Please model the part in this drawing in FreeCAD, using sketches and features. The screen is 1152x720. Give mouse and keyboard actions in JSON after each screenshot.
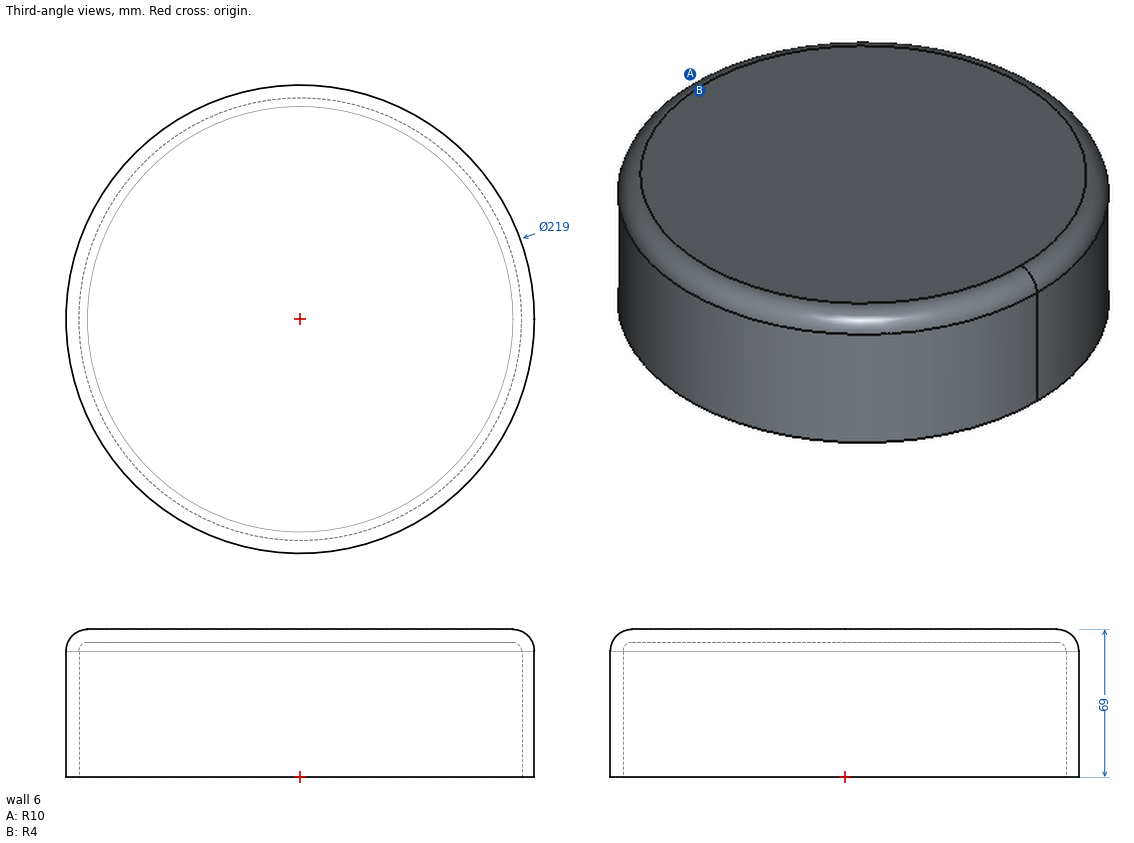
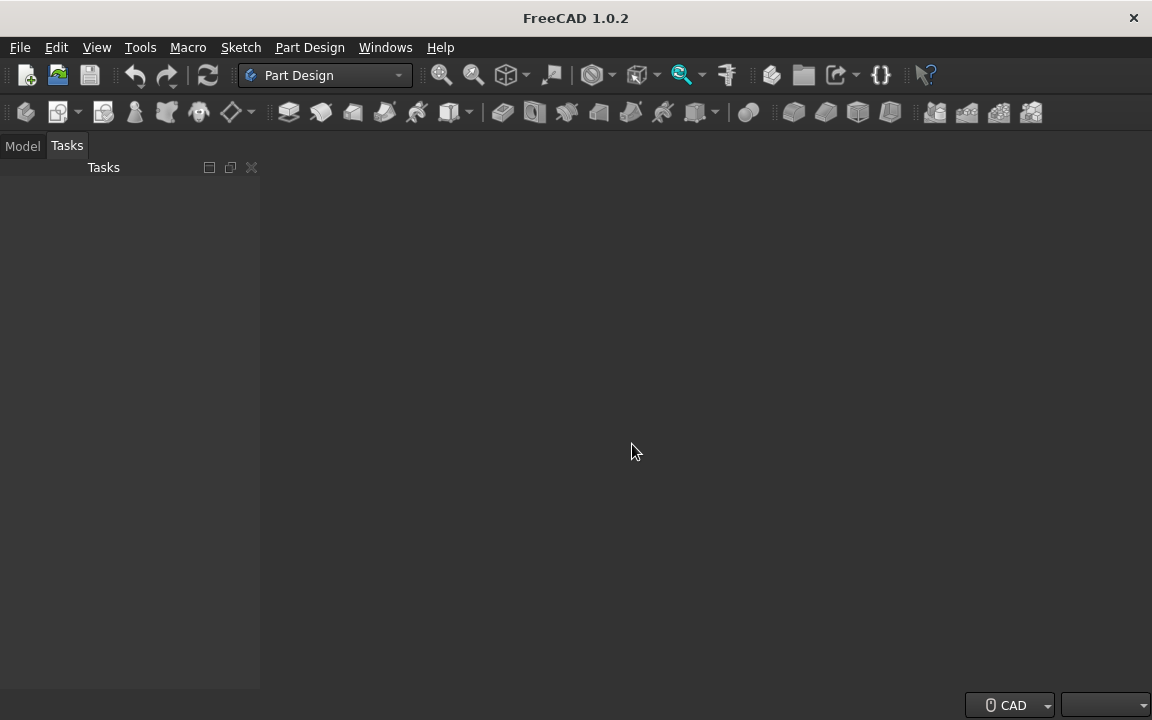
{"action": "key", "text": "ctrl+n"}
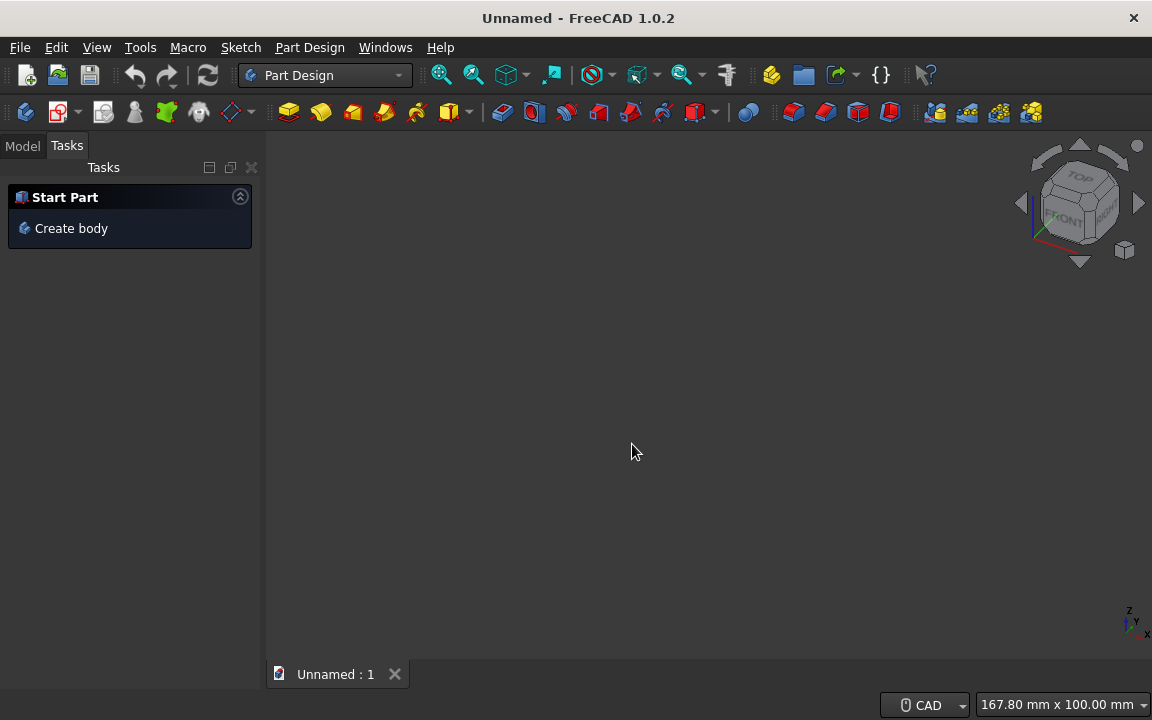
{"action": "left_click", "coordinate": [58, 112]}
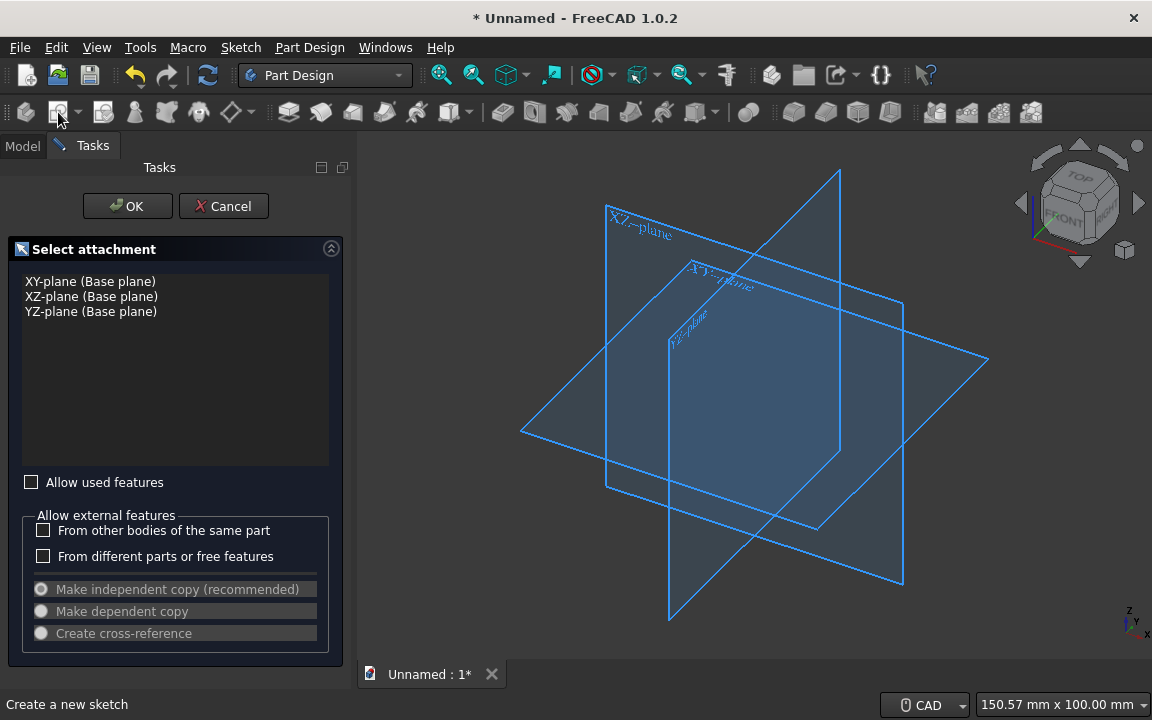
{"action": "left_click", "coordinate": [82, 282]}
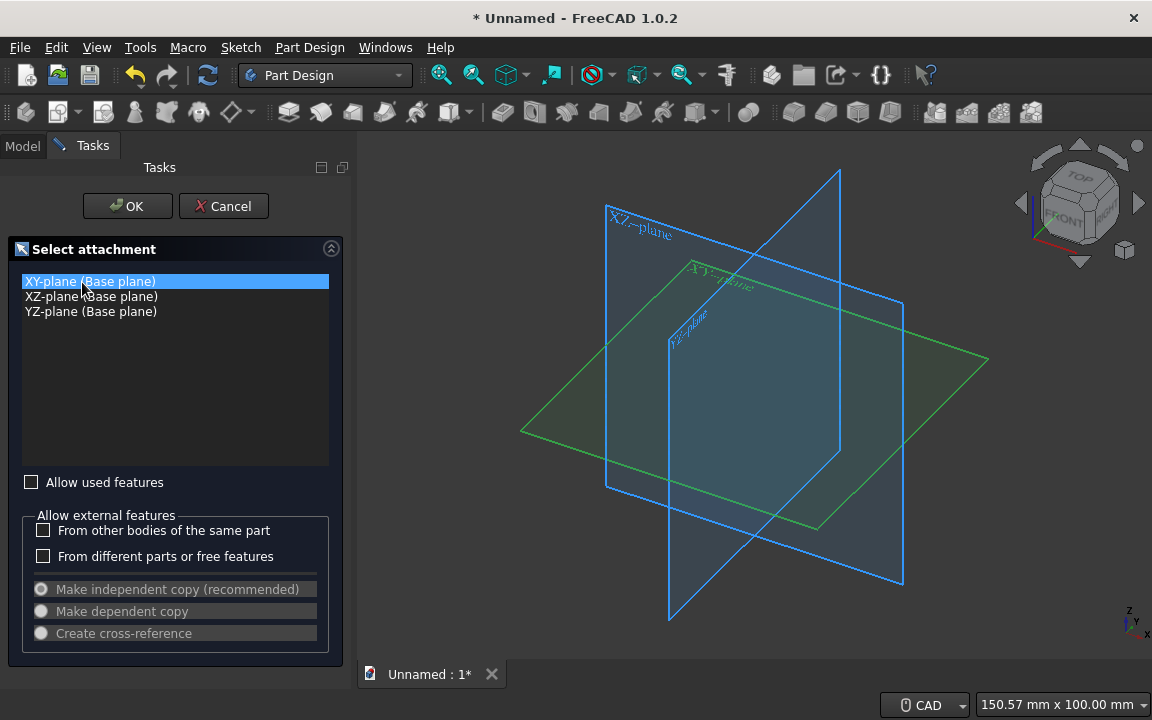
{"action": "left_click", "coordinate": [128, 206]}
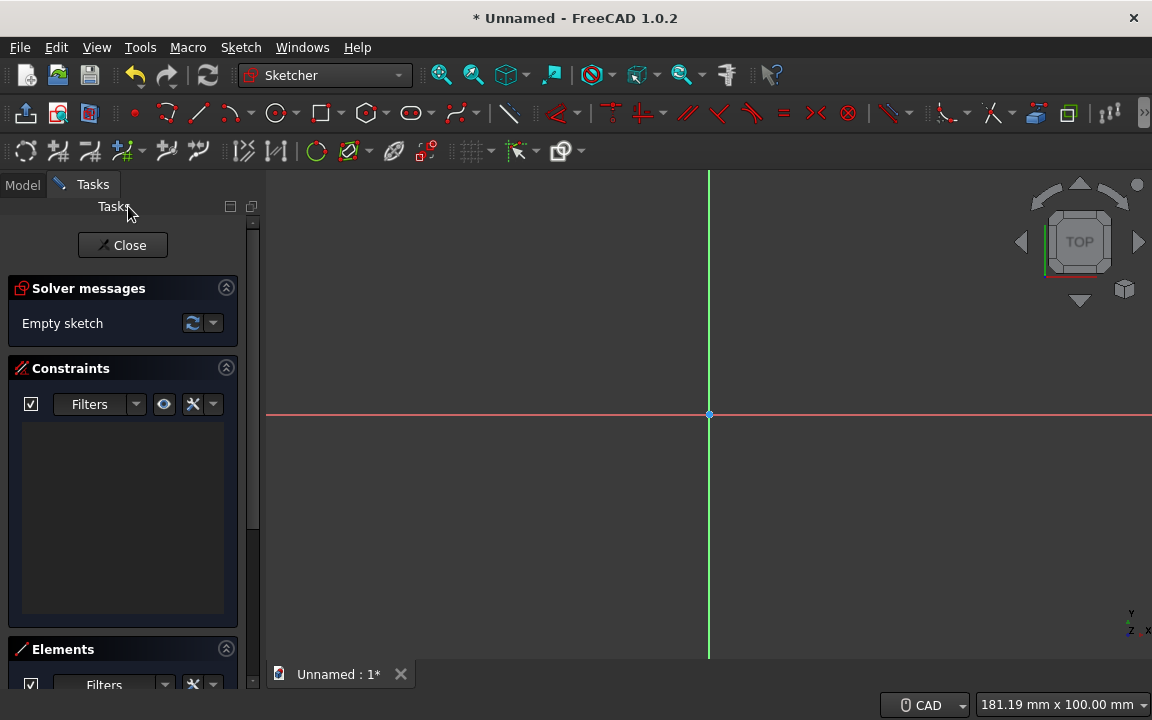
{"action": "scroll", "coordinate": [611, 414], "scroll_direction": "down", "scroll_amount": 6}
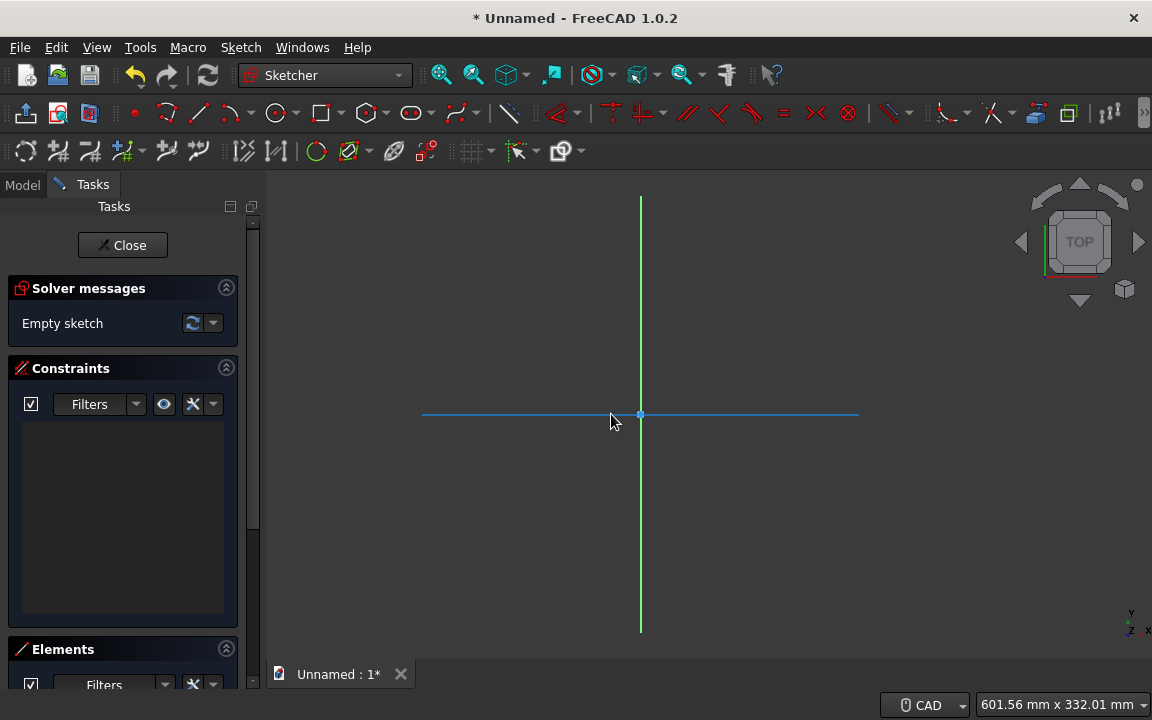
{"action": "key", "text": "g c"}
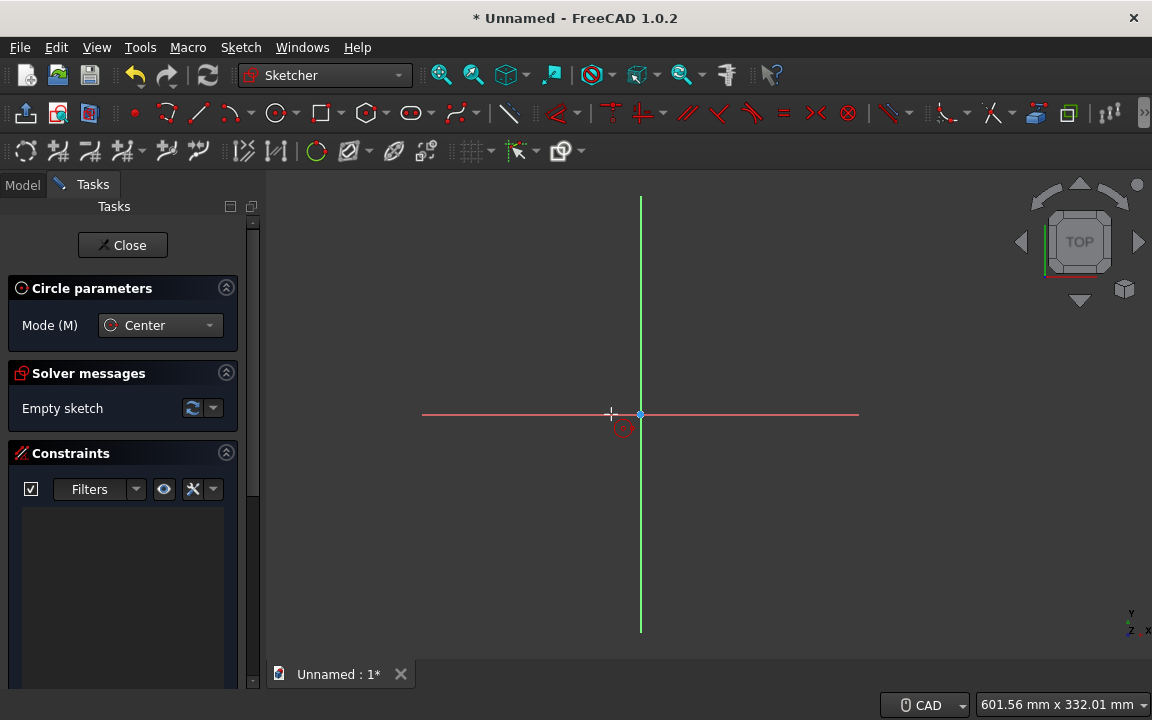
{"action": "left_click", "coordinate": [641, 414]}
{"action": "left_click", "coordinate": [755, 300]}
{"action": "key", "text": "Escape"}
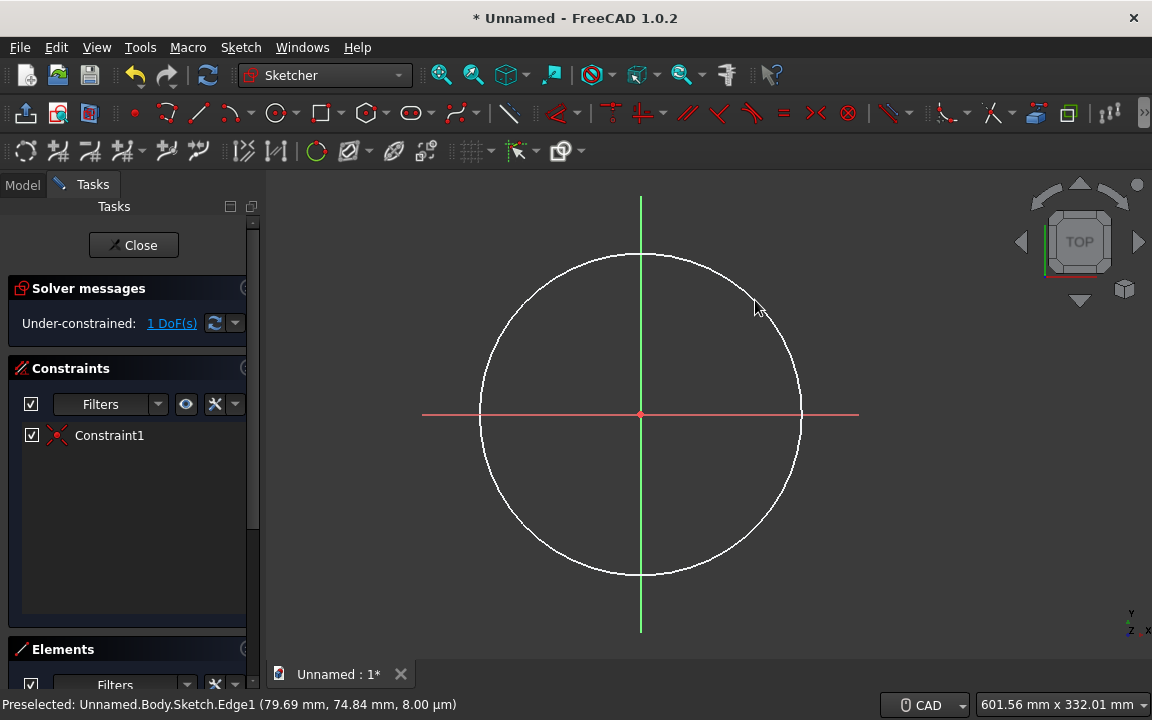
{"action": "key", "text": "d"}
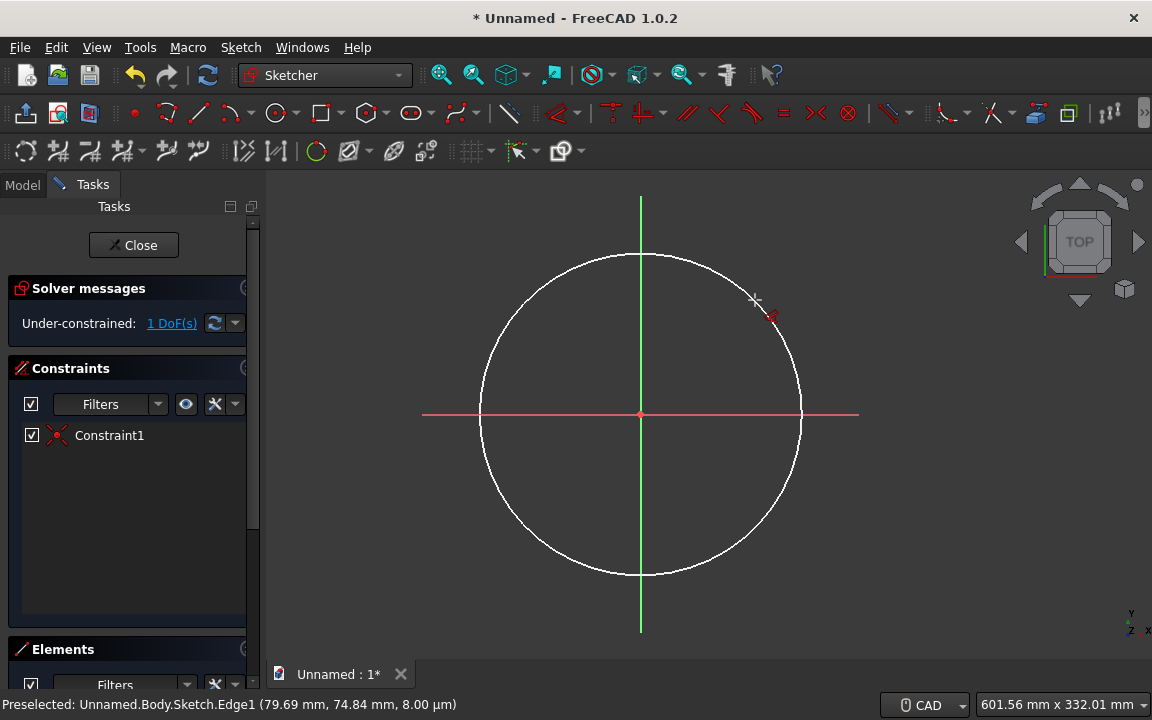
{"action": "left_click", "coordinate": [754, 300]}
{"action": "left_click", "coordinate": [776, 277]}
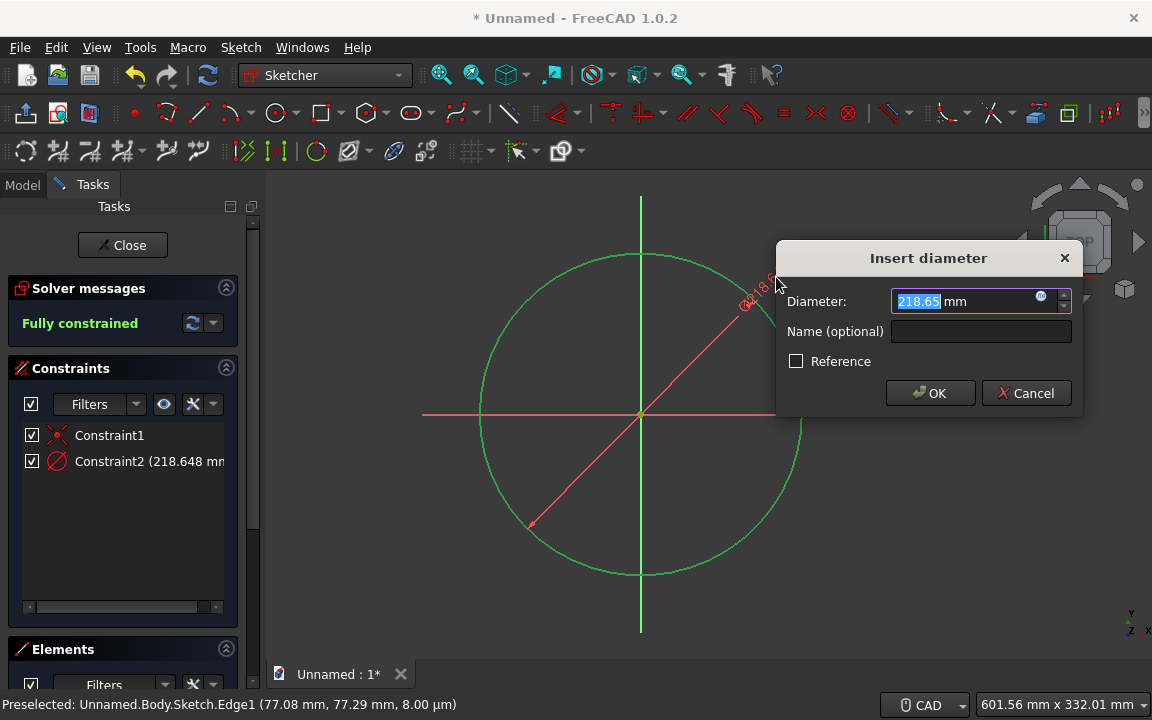
{"action": "type", "text": "219"}
{"action": "key", "text": "Return"}
{"action": "key", "text": "Escape"}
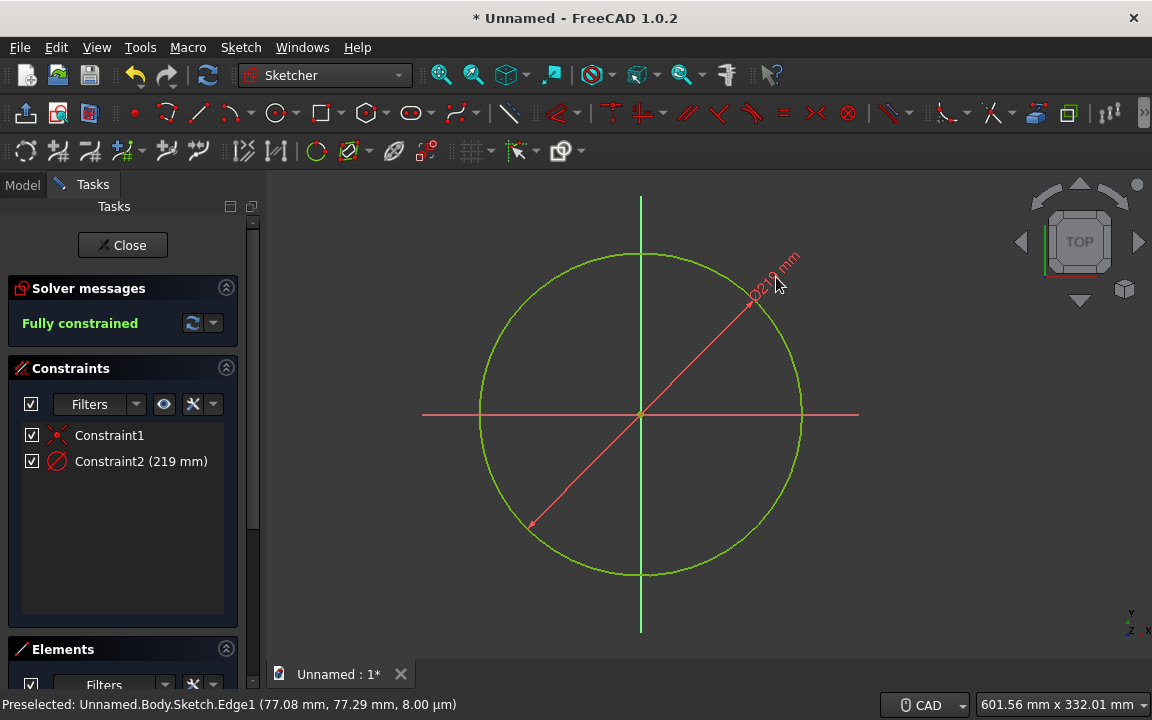
{"action": "left_click", "coordinate": [123, 245]}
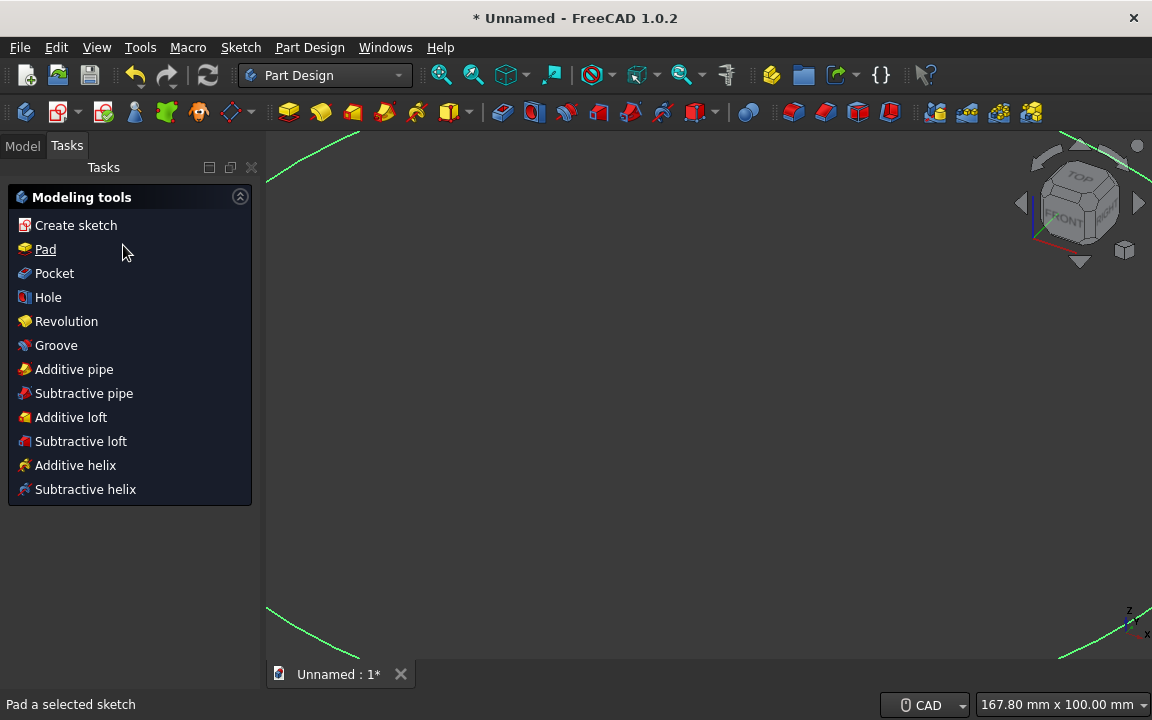
{"action": "left_click", "coordinate": [290, 112]}